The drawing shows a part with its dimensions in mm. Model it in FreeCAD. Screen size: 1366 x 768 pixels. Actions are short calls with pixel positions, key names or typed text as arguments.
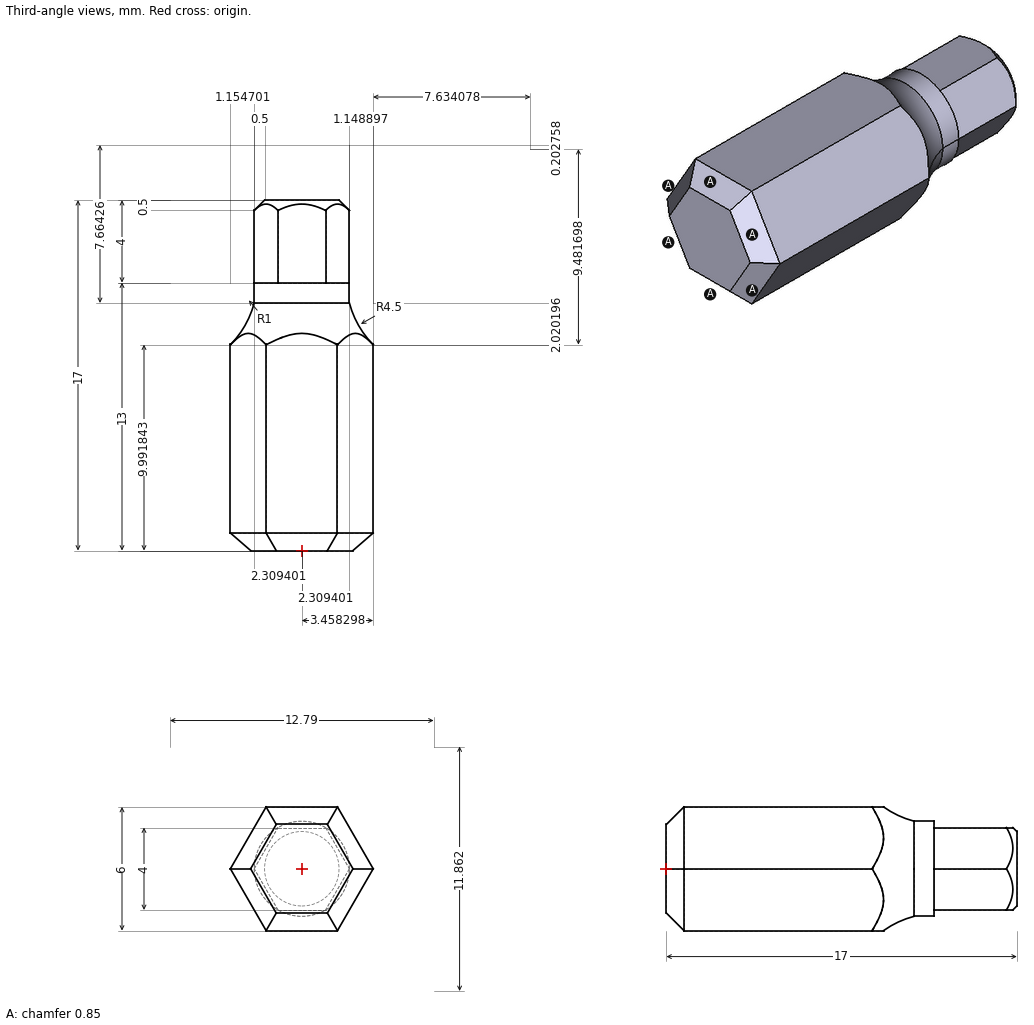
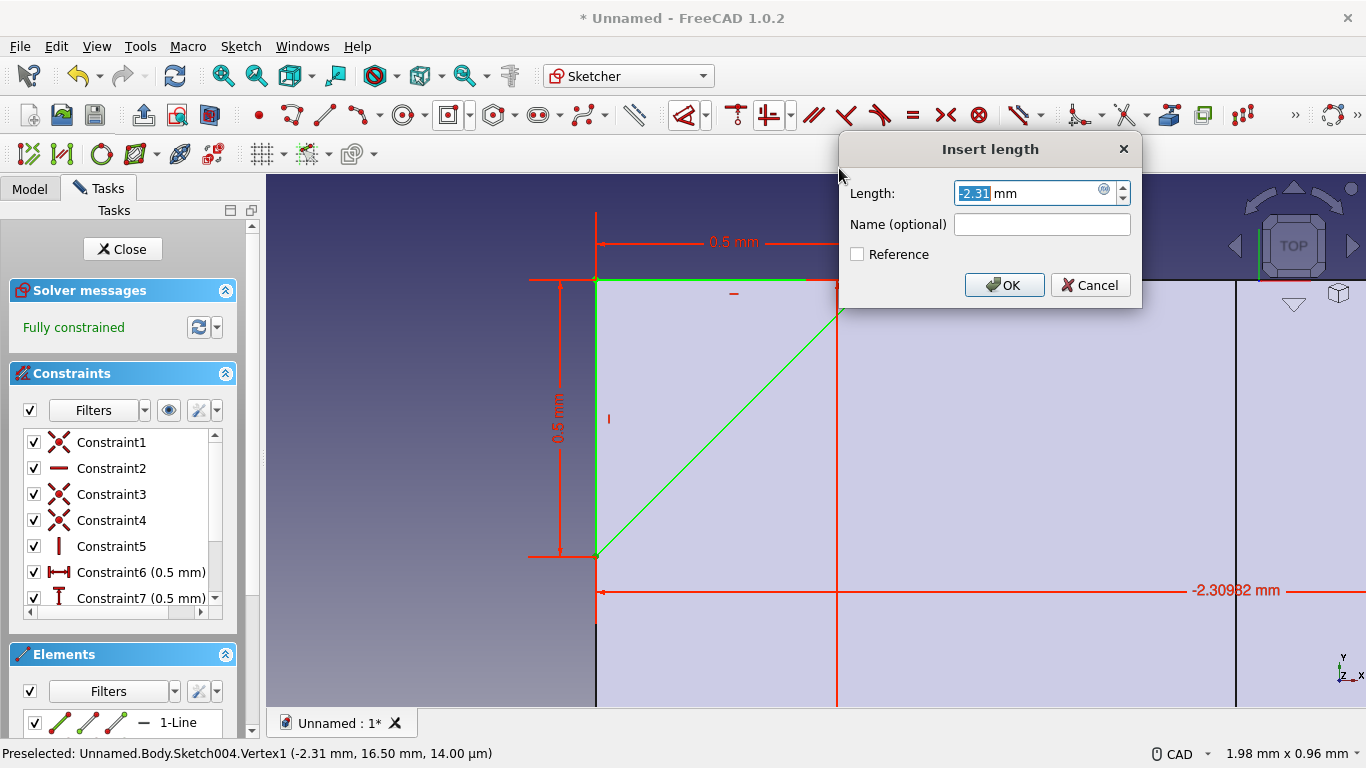
text(-2.309401)
key(Return)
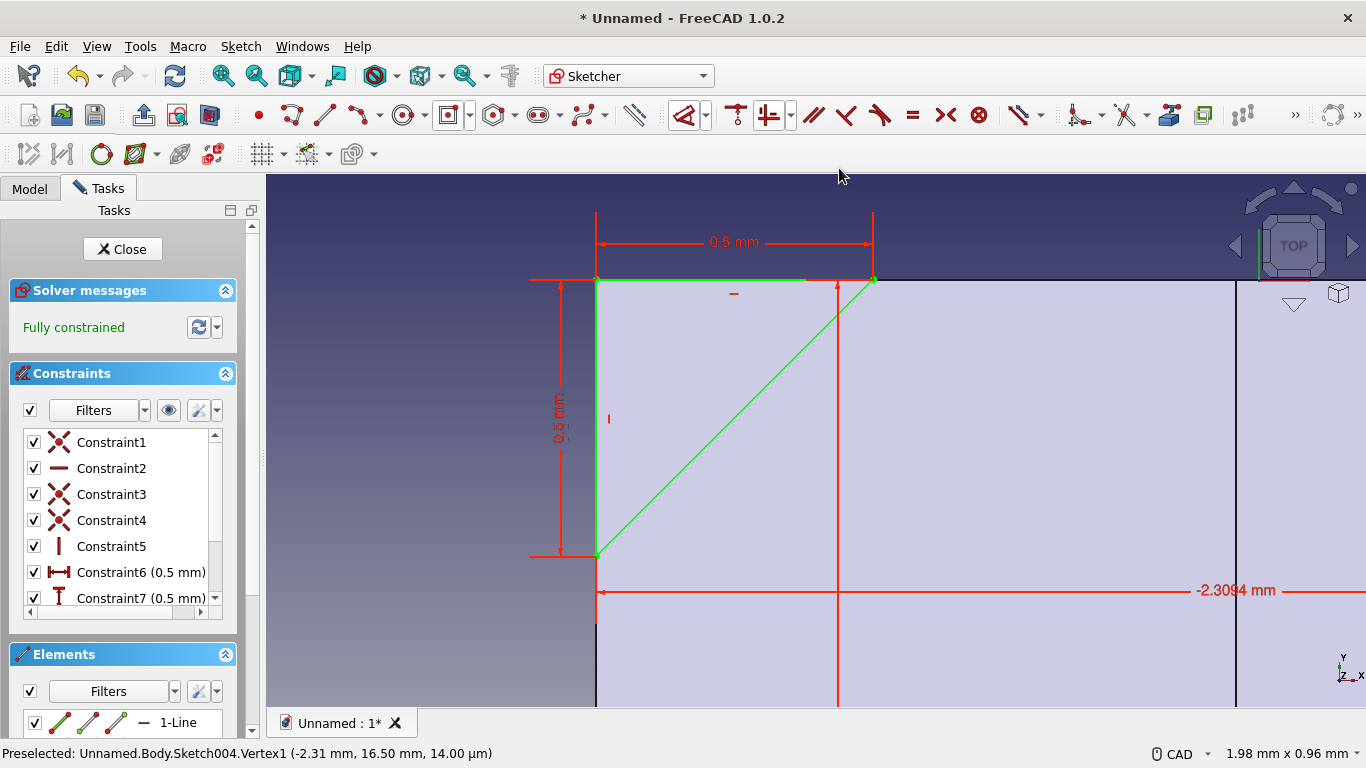
click(123, 249)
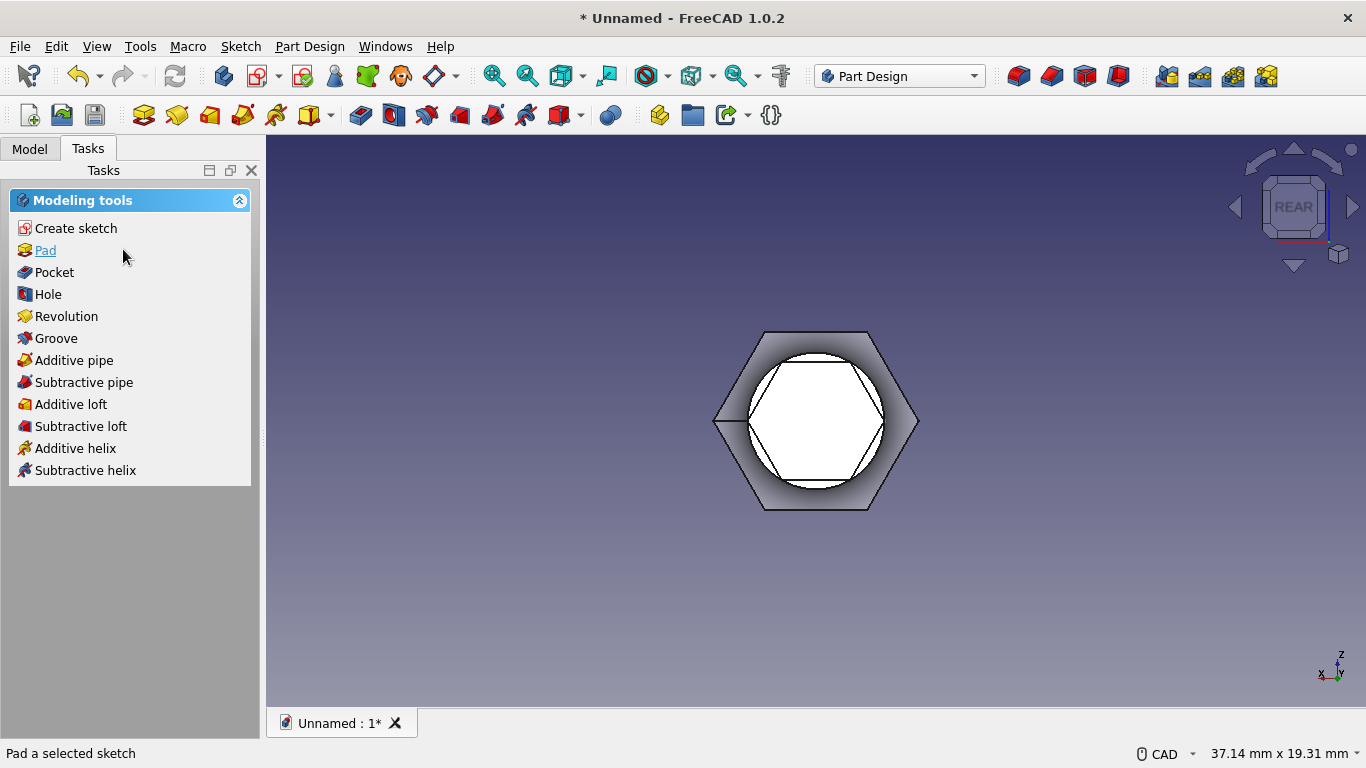
click(427, 116)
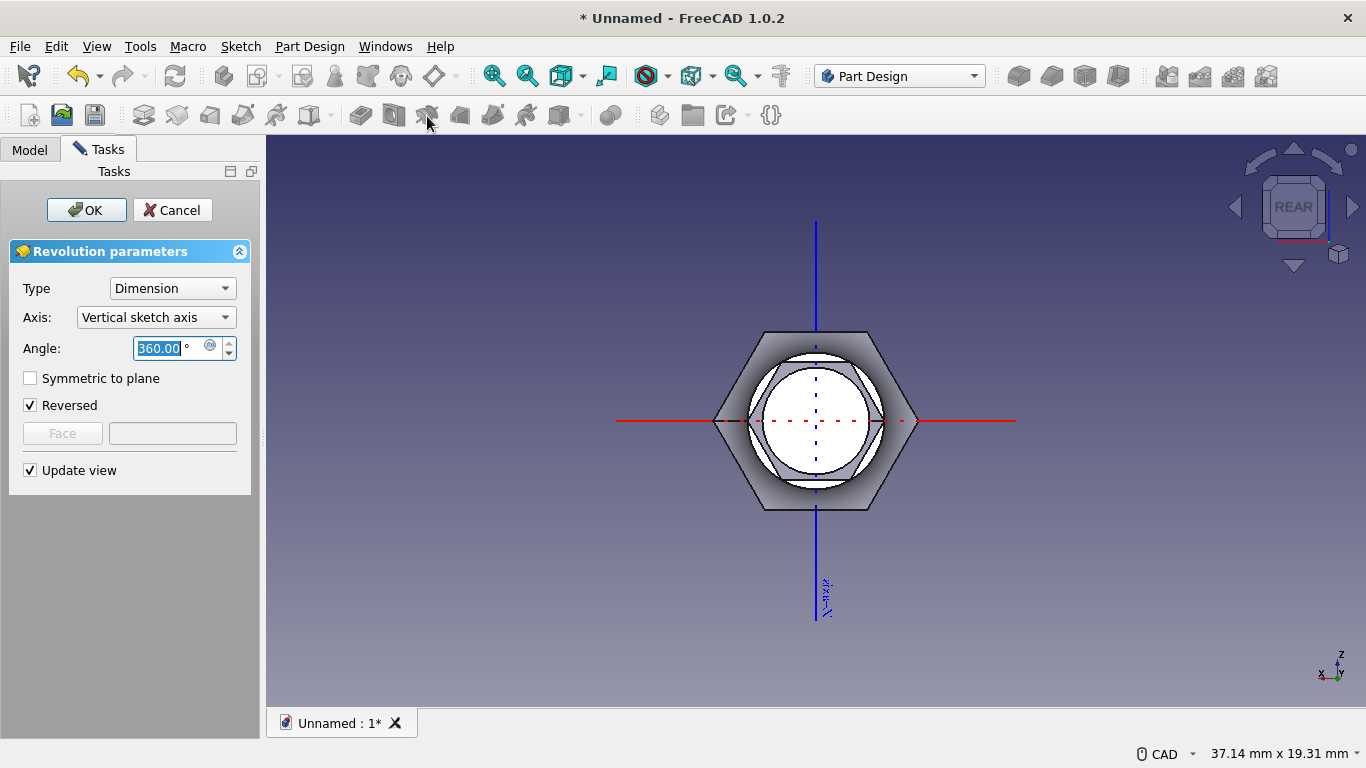
click(87, 210)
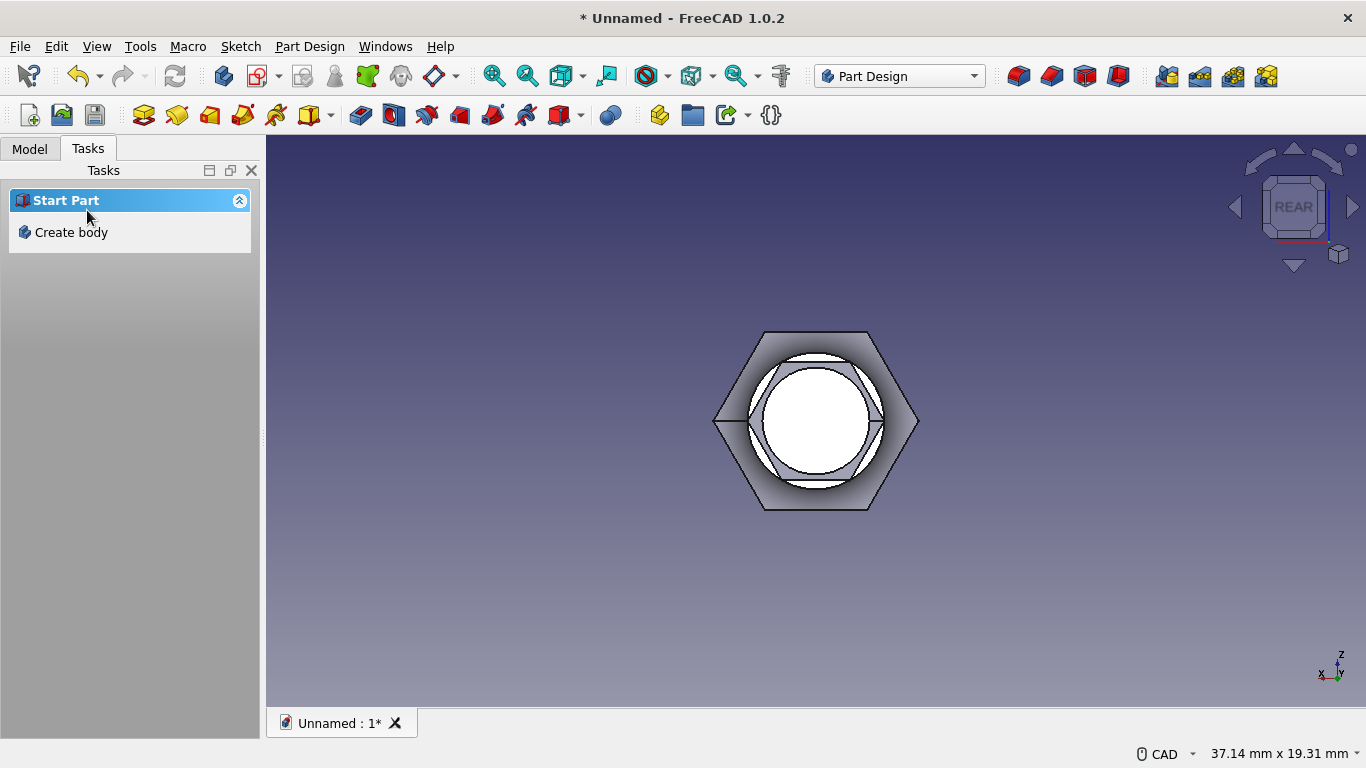
key(0)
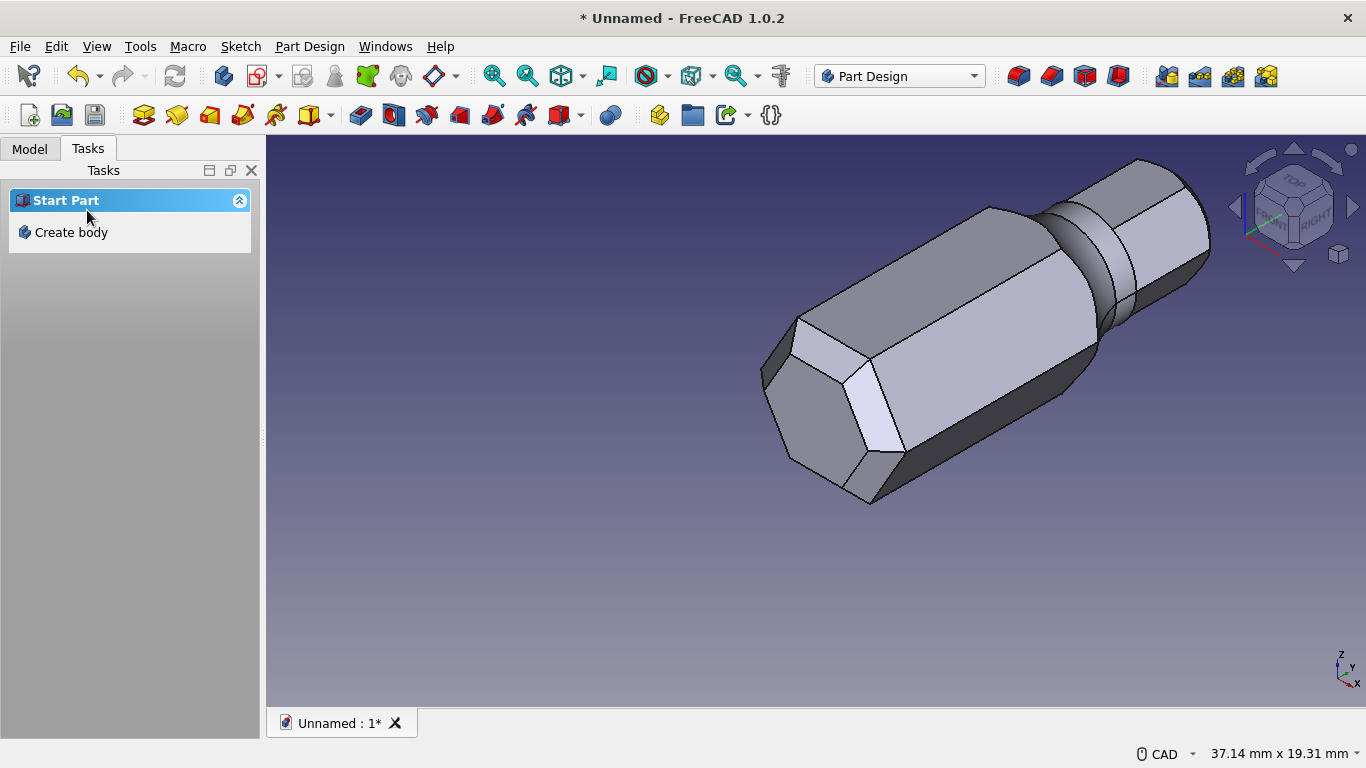
click(495, 76)